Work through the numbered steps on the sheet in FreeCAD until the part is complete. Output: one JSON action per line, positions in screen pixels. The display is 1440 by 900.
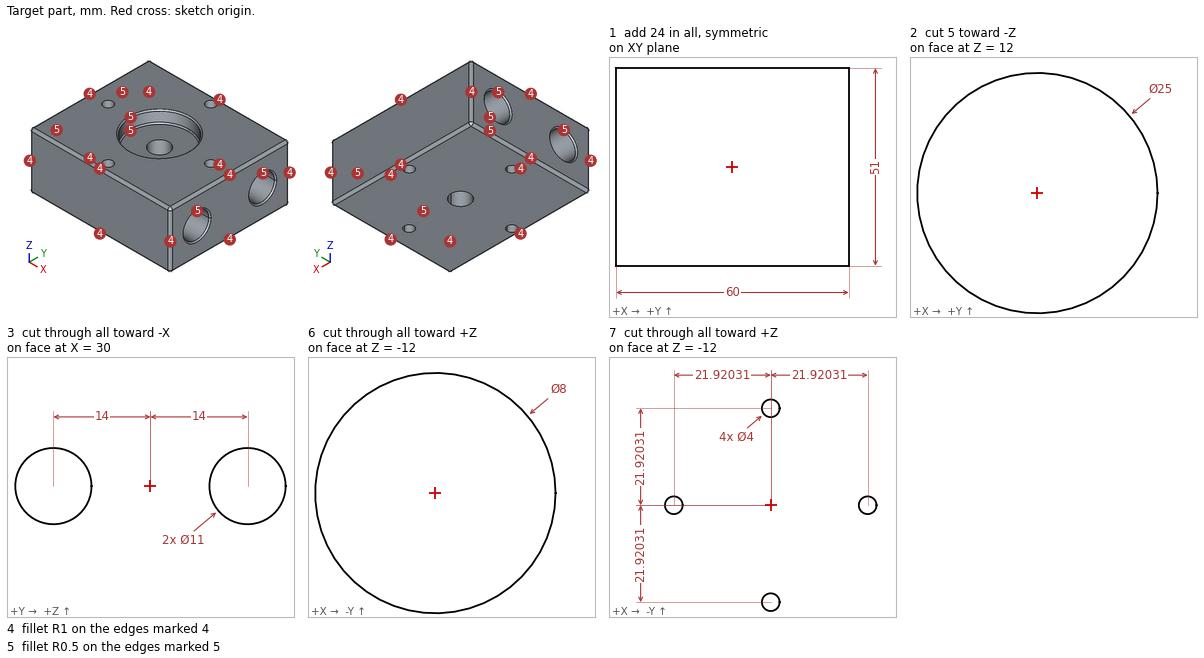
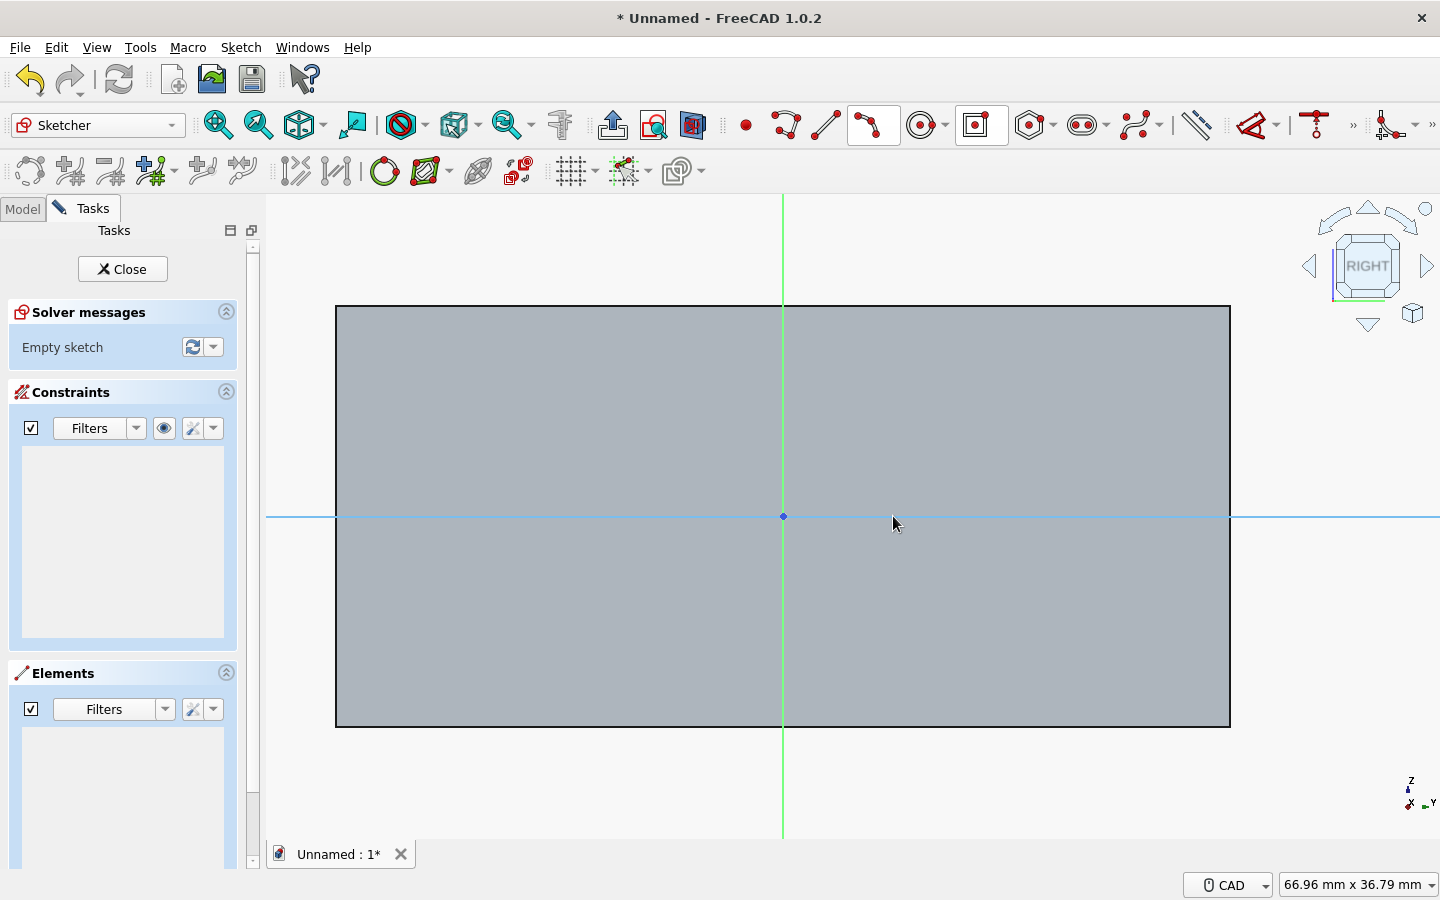
{"action": "left_click", "coordinate": [922, 126]}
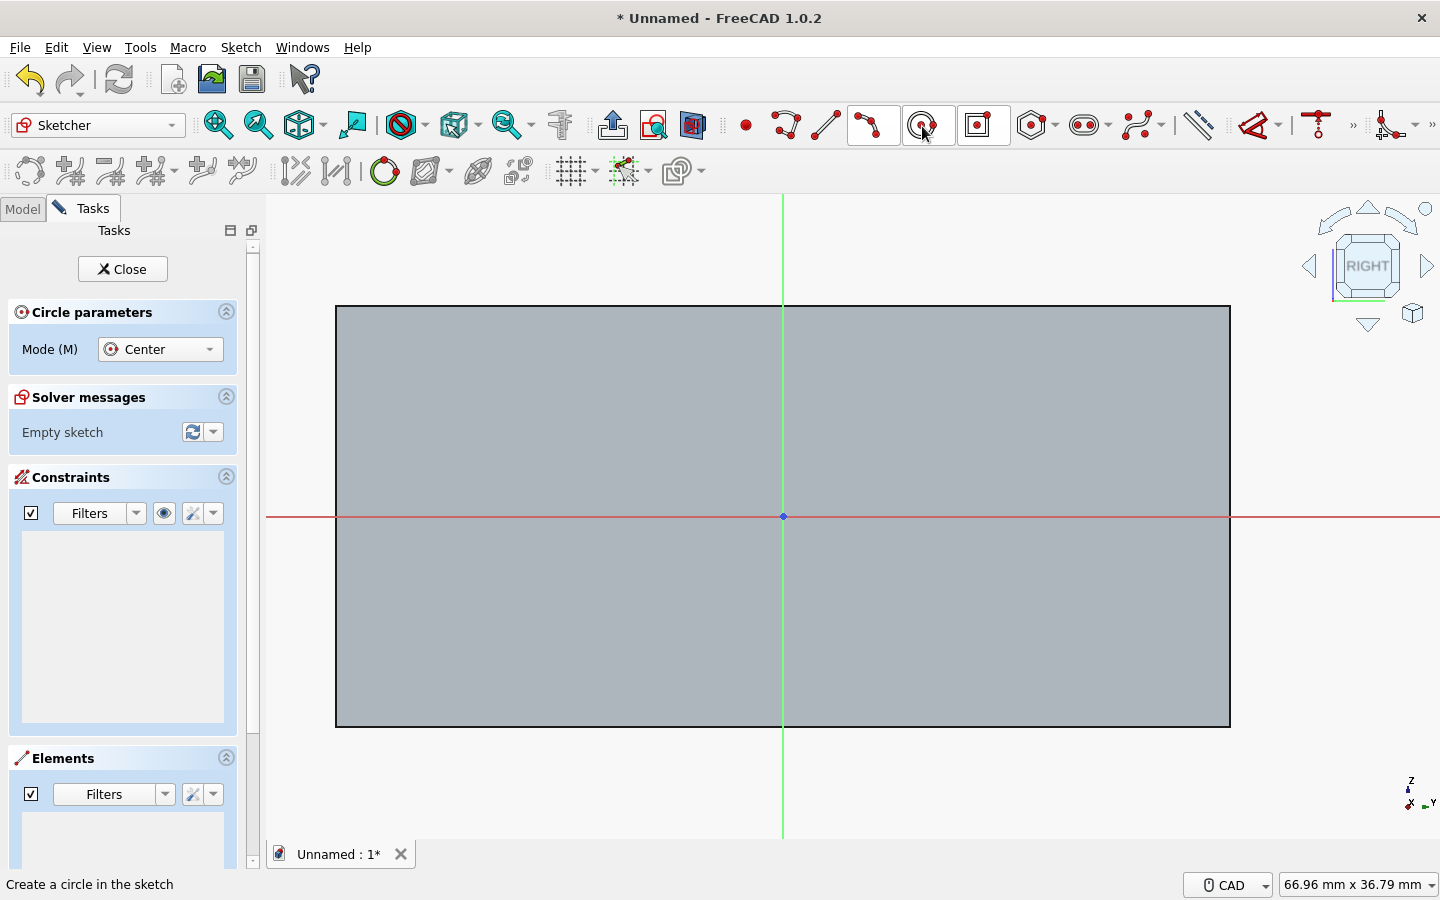
{"action": "left_click", "coordinate": [1029, 516]}
{"action": "left_click", "coordinate": [1097, 448]}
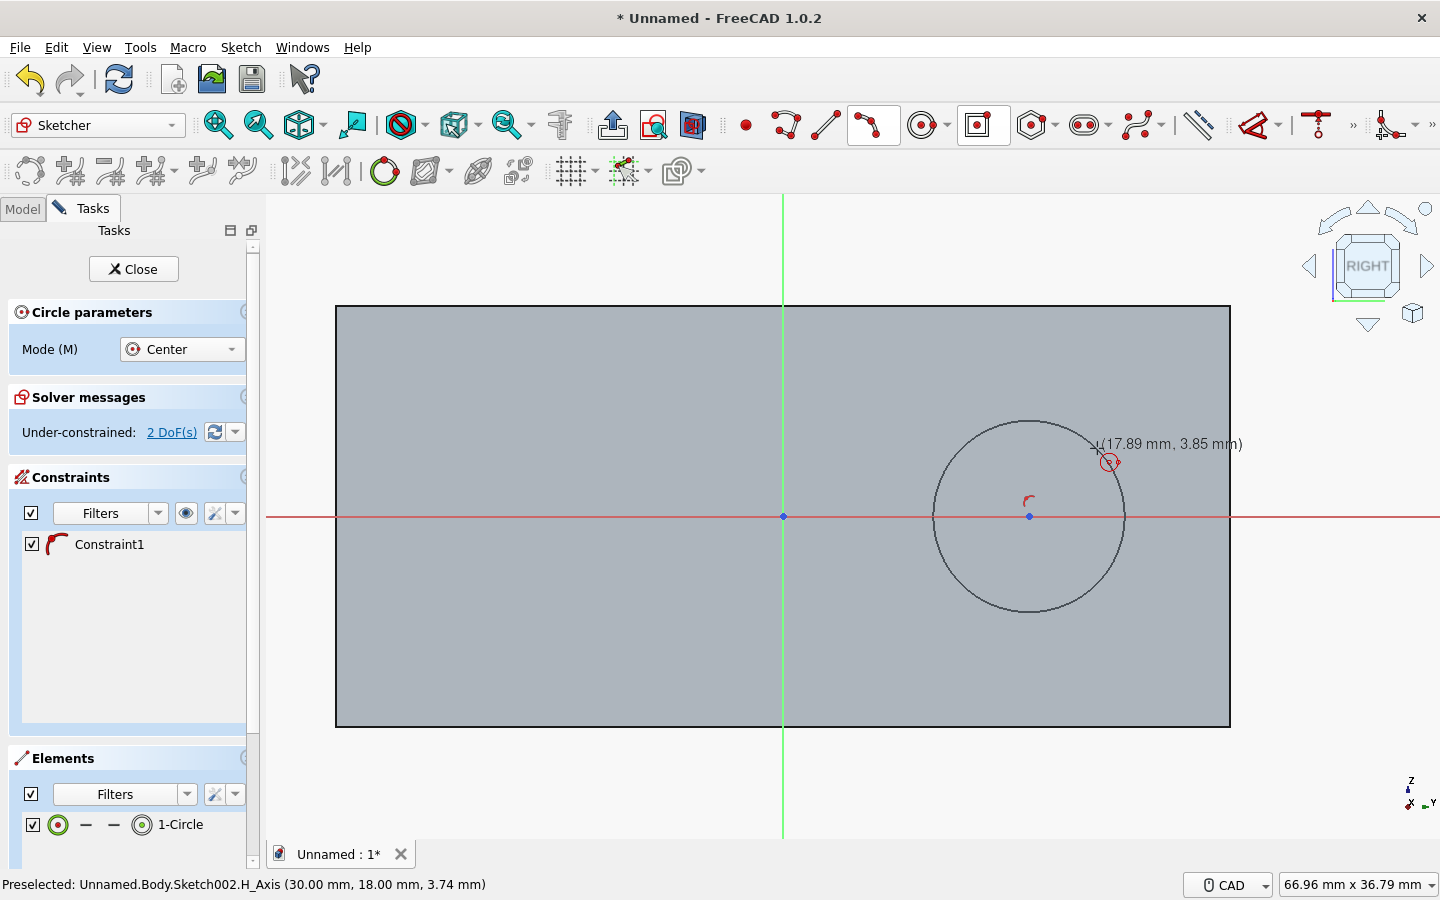
{"action": "left_click", "coordinate": [538, 516]}
{"action": "left_click", "coordinate": [606, 448]}
{"action": "key", "text": "Escape"}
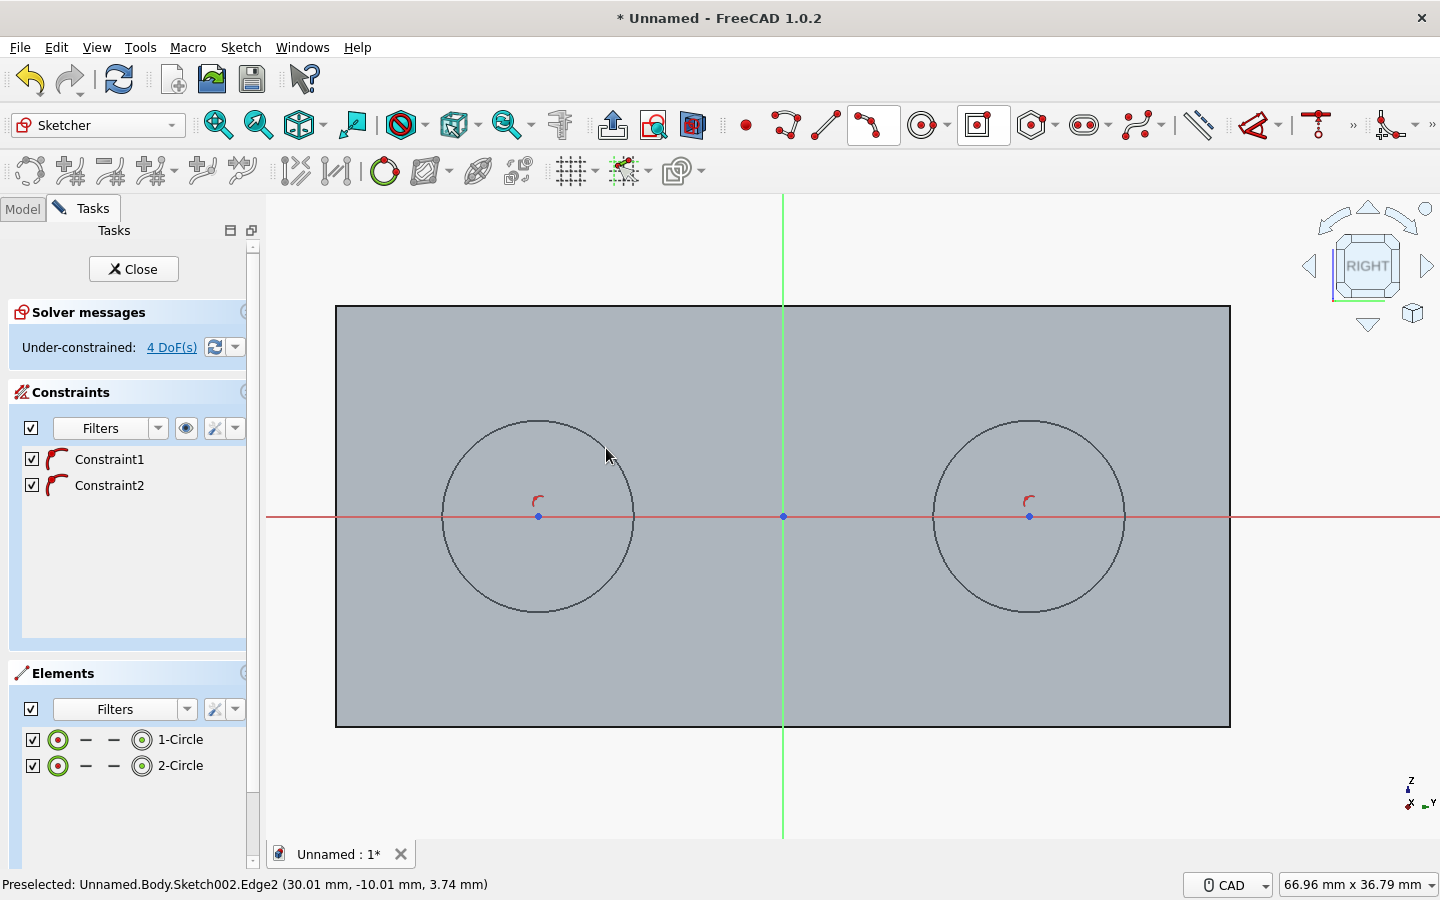
{"action": "left_click", "coordinate": [1097, 449]}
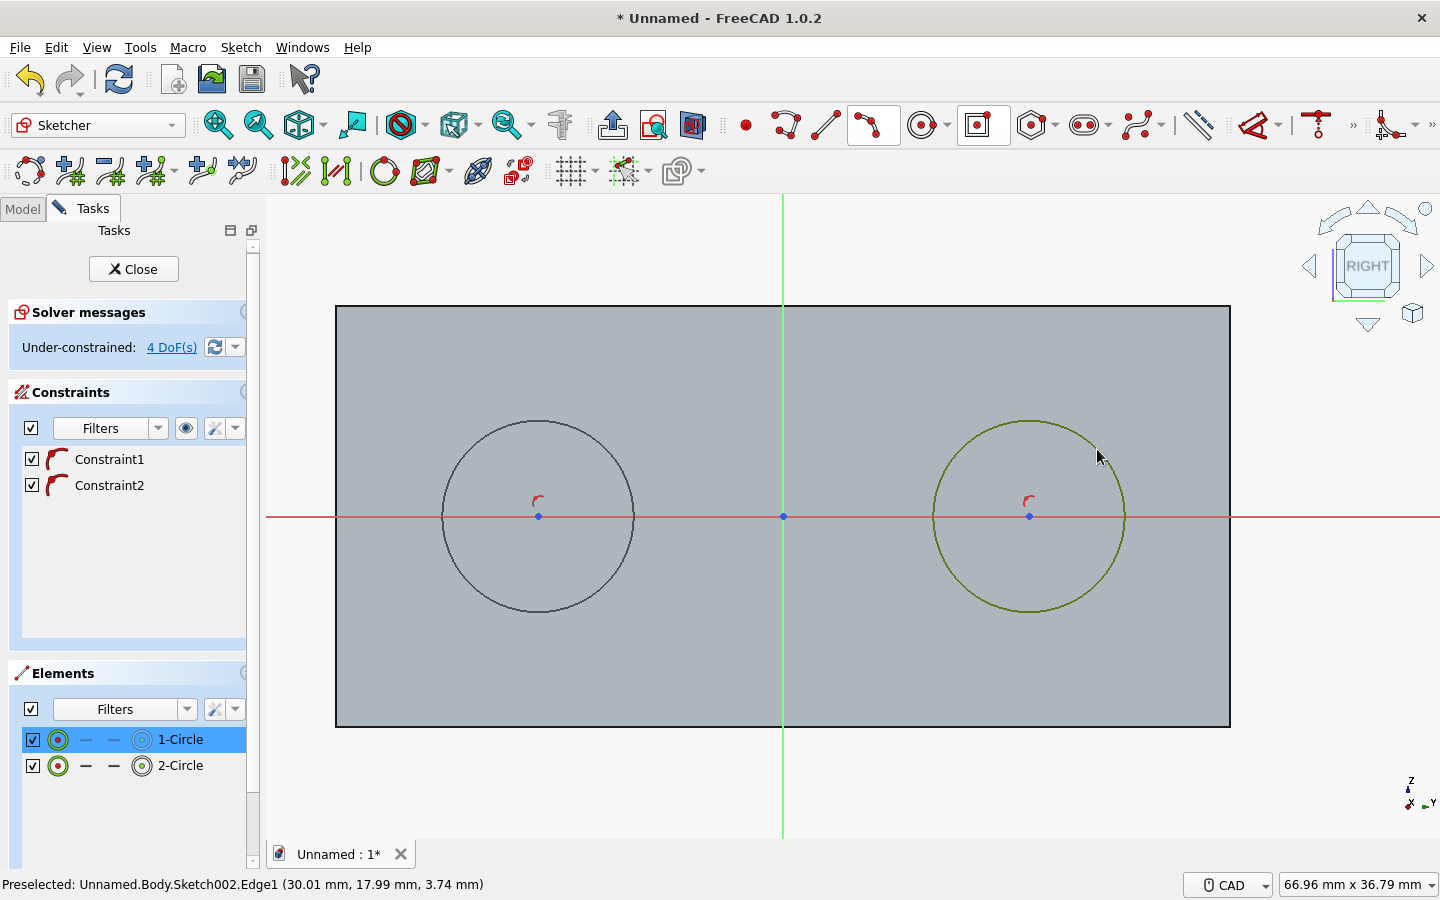
{"action": "left_click", "coordinate": [606, 449]}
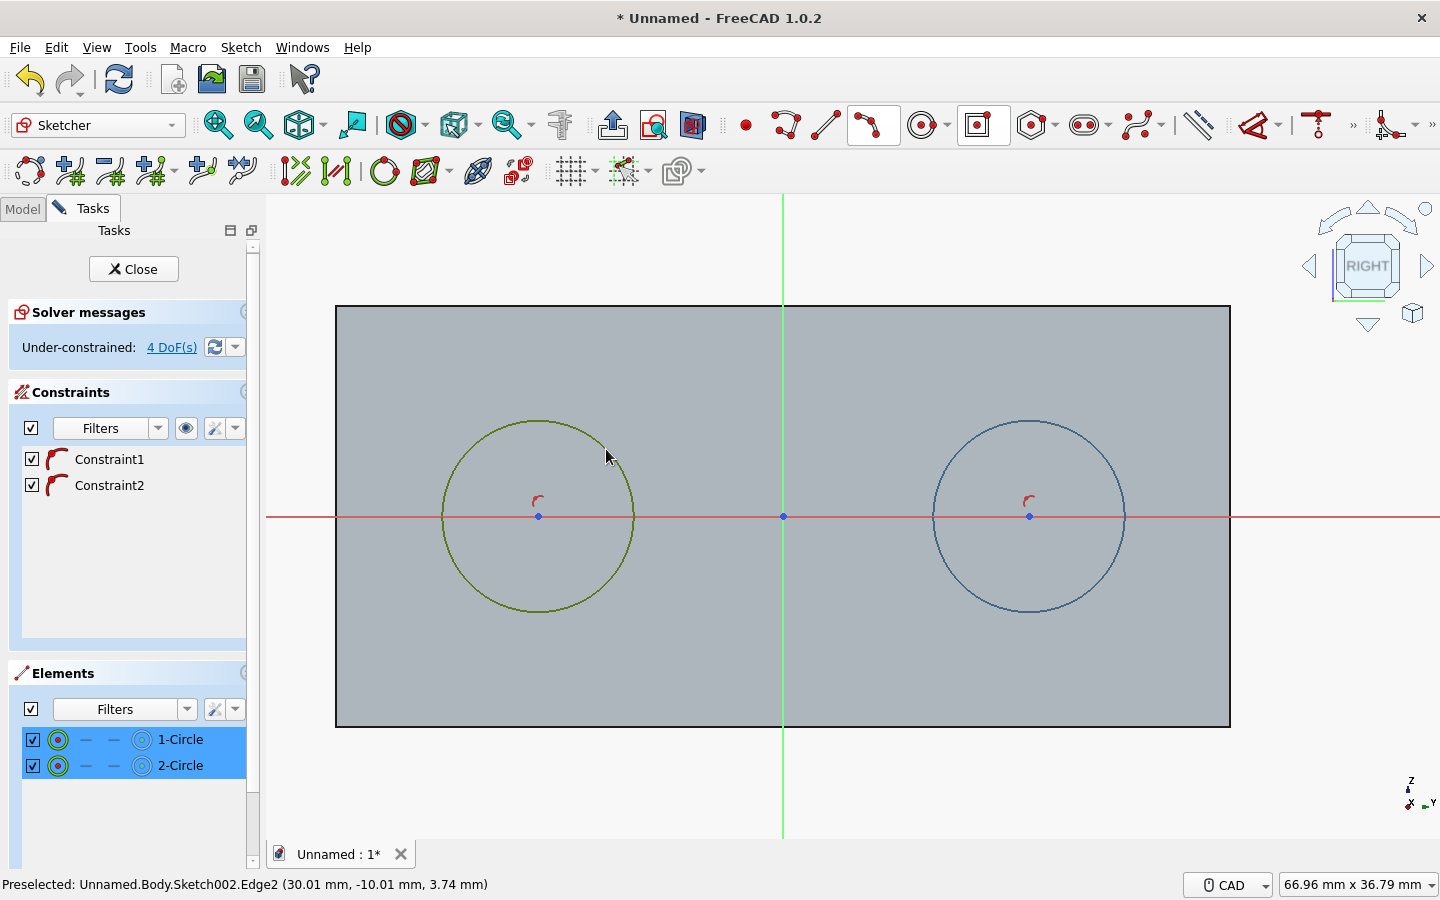
{"action": "key", "text": "e"}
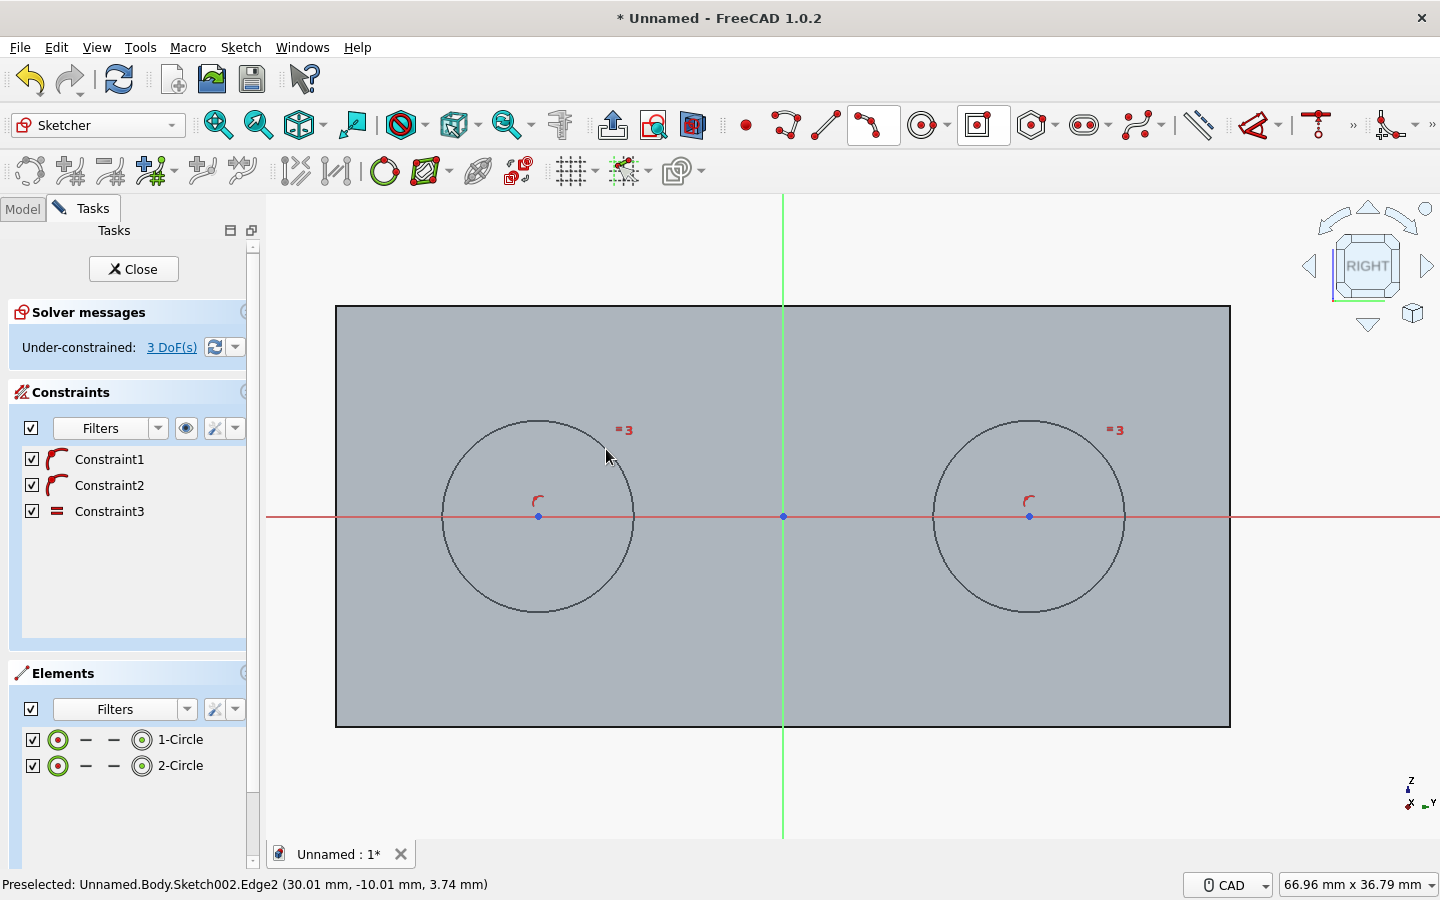
{"action": "left_click", "coordinate": [1254, 126]}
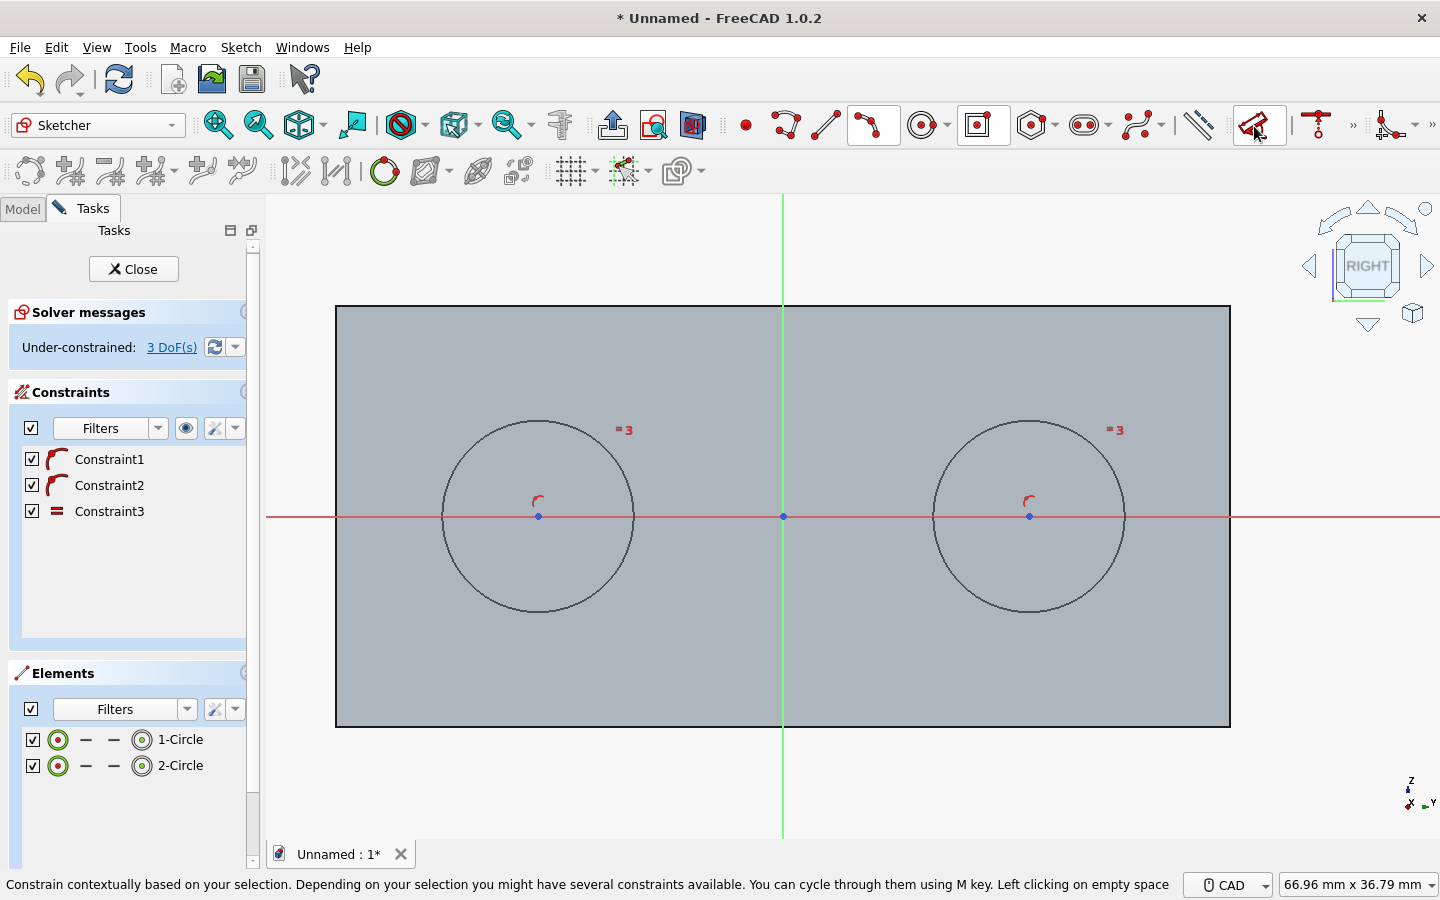
{"action": "left_click", "coordinate": [1097, 449]}
{"action": "left_click", "coordinate": [1120, 426]}